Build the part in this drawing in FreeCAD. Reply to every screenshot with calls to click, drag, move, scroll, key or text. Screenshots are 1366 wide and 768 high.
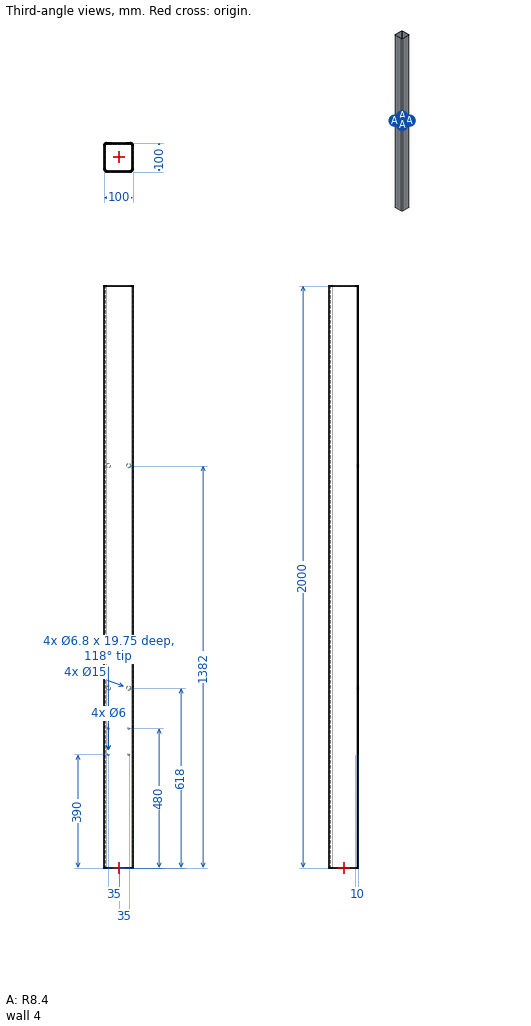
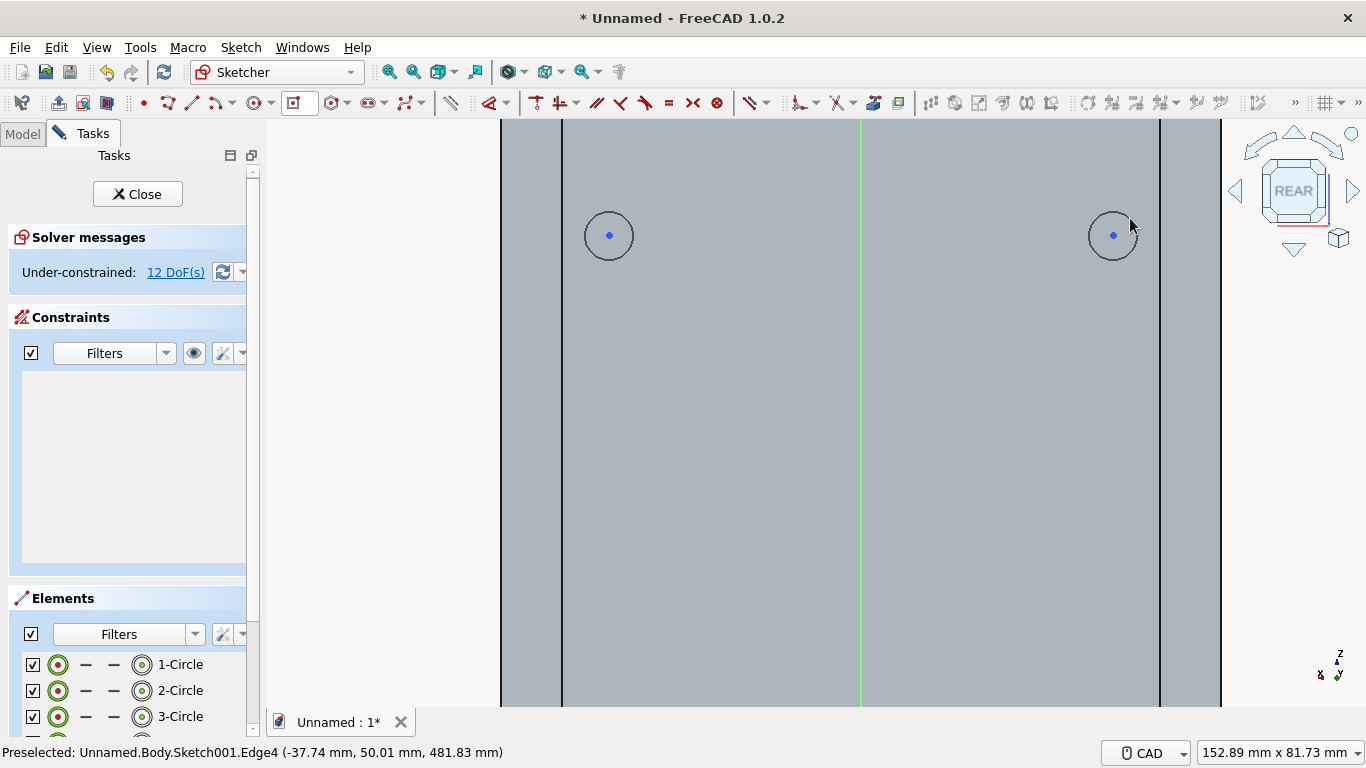
scroll(610, 236, down, 3)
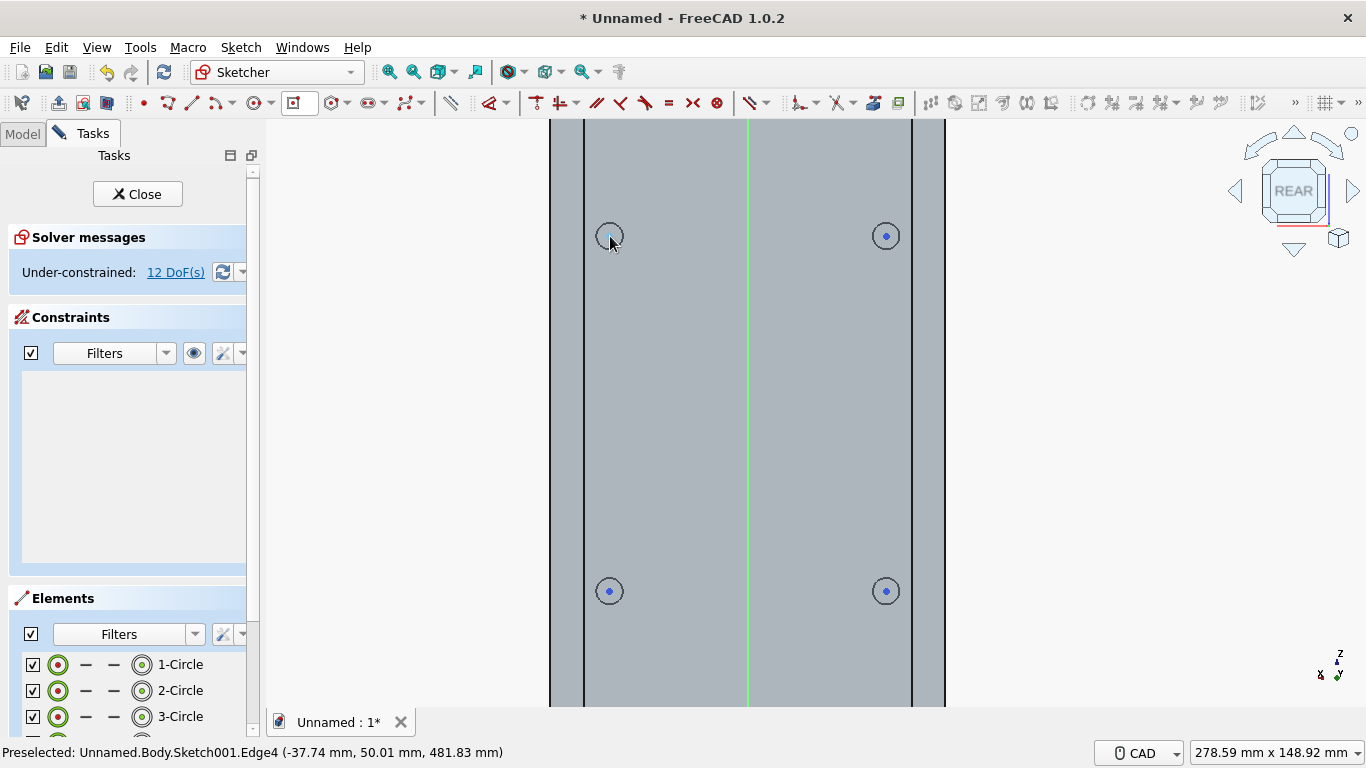
click(895, 582)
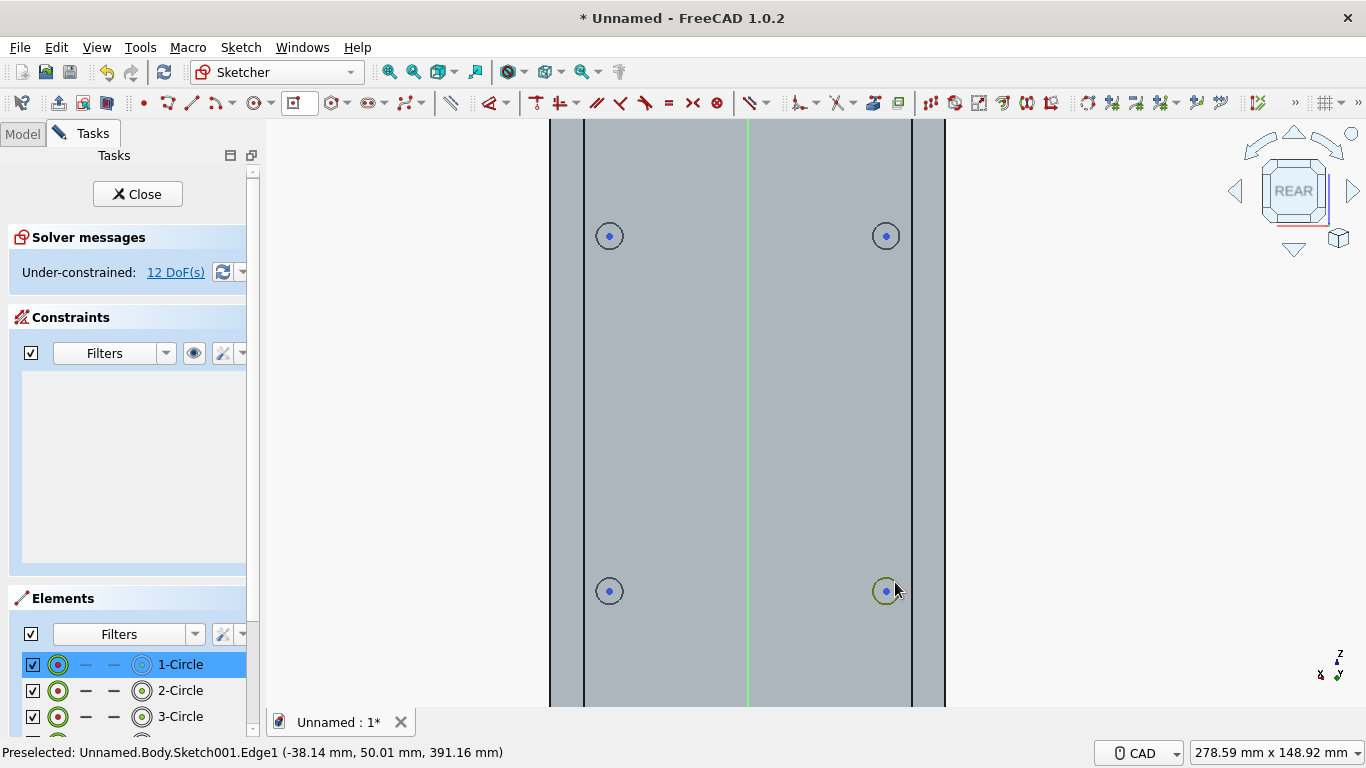
click(619, 582)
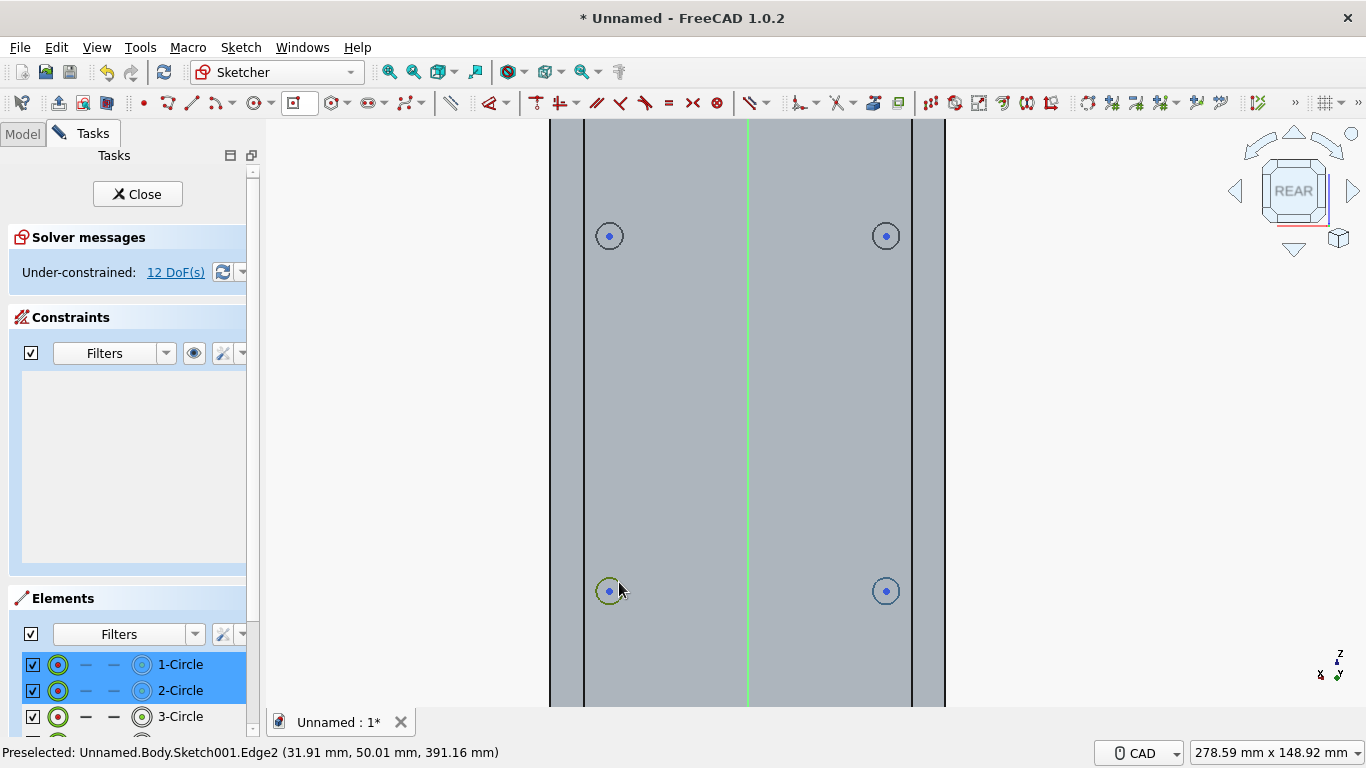
click(619, 227)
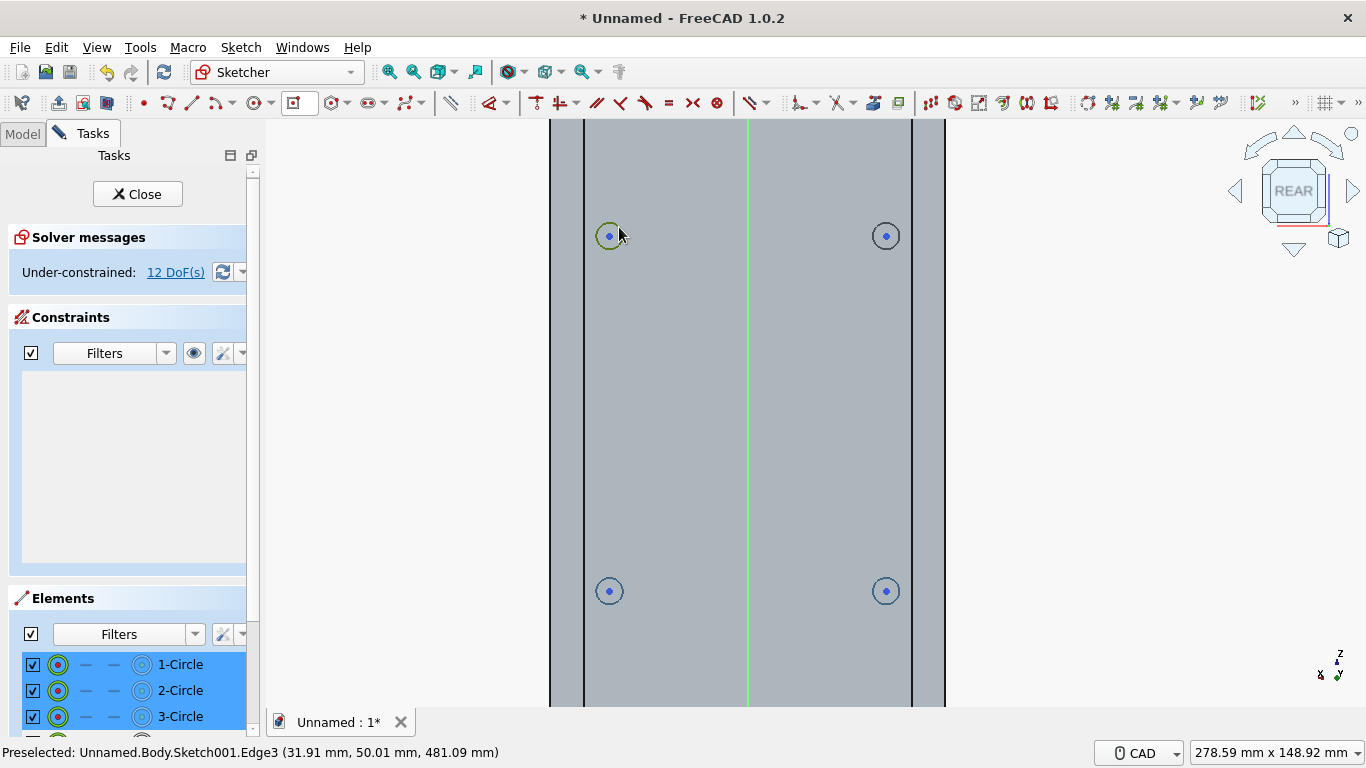
click(895, 227)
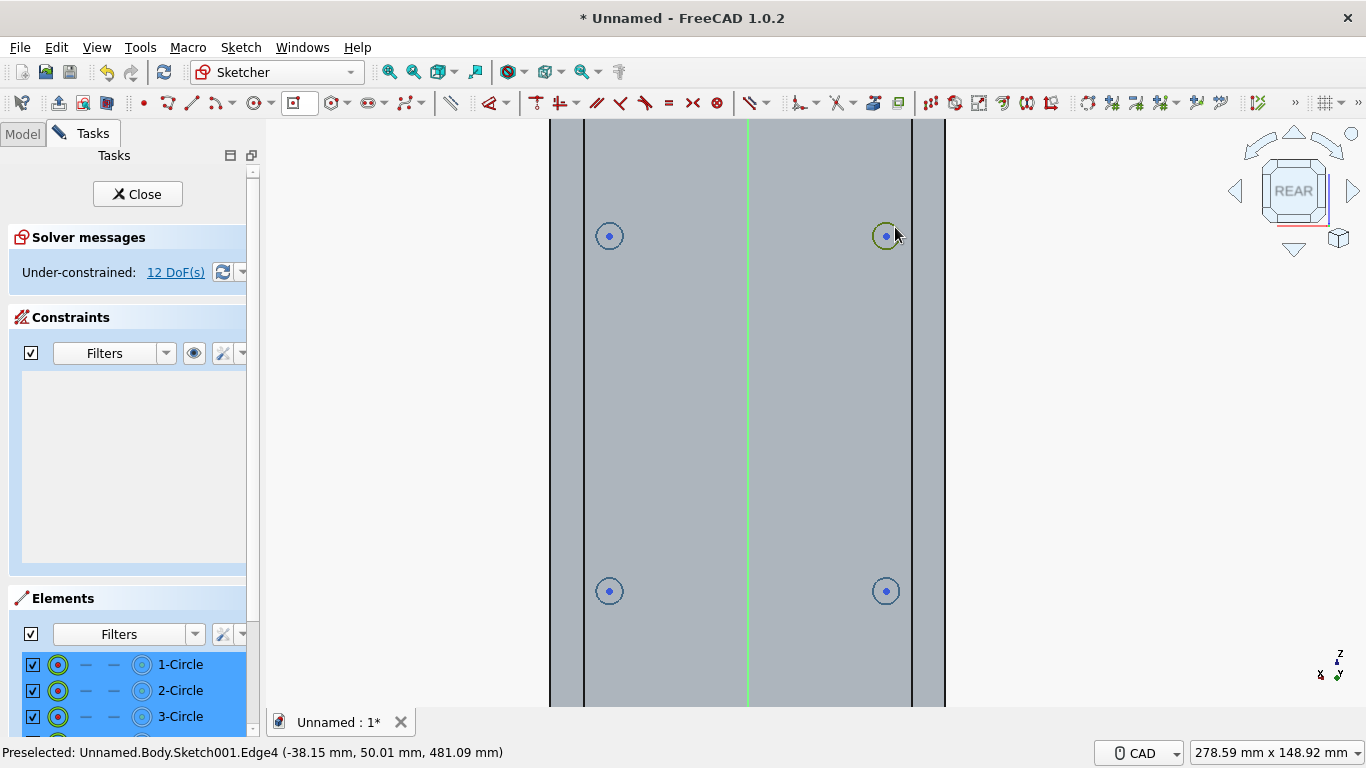
click(670, 104)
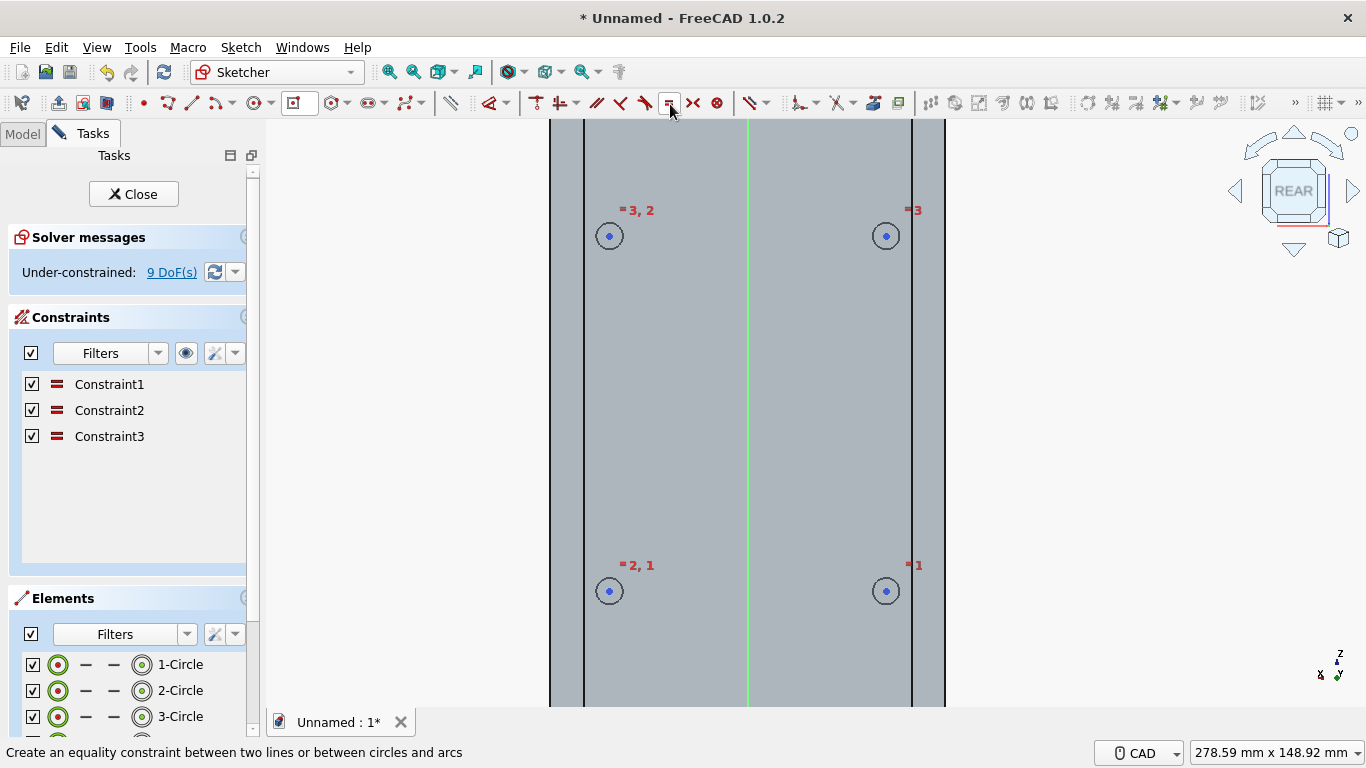
click(886, 591)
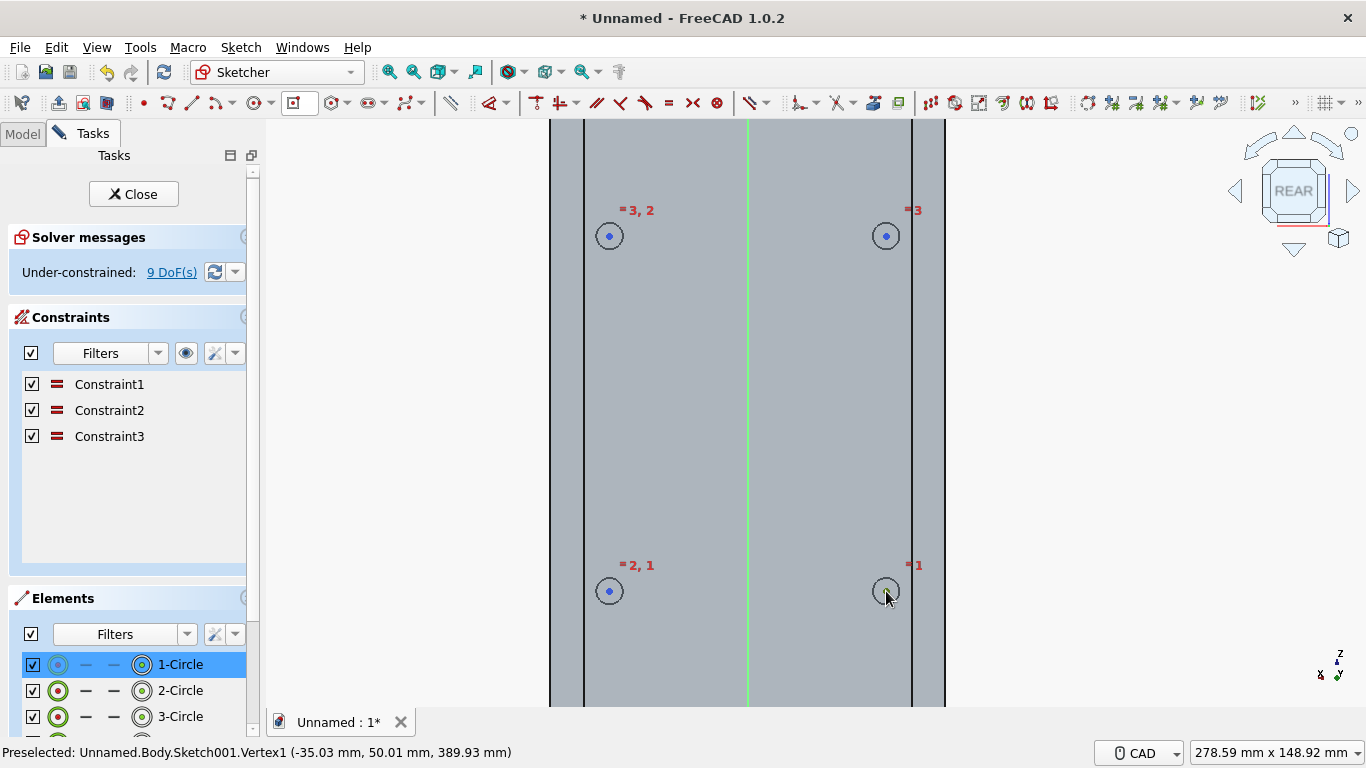
click(610, 591)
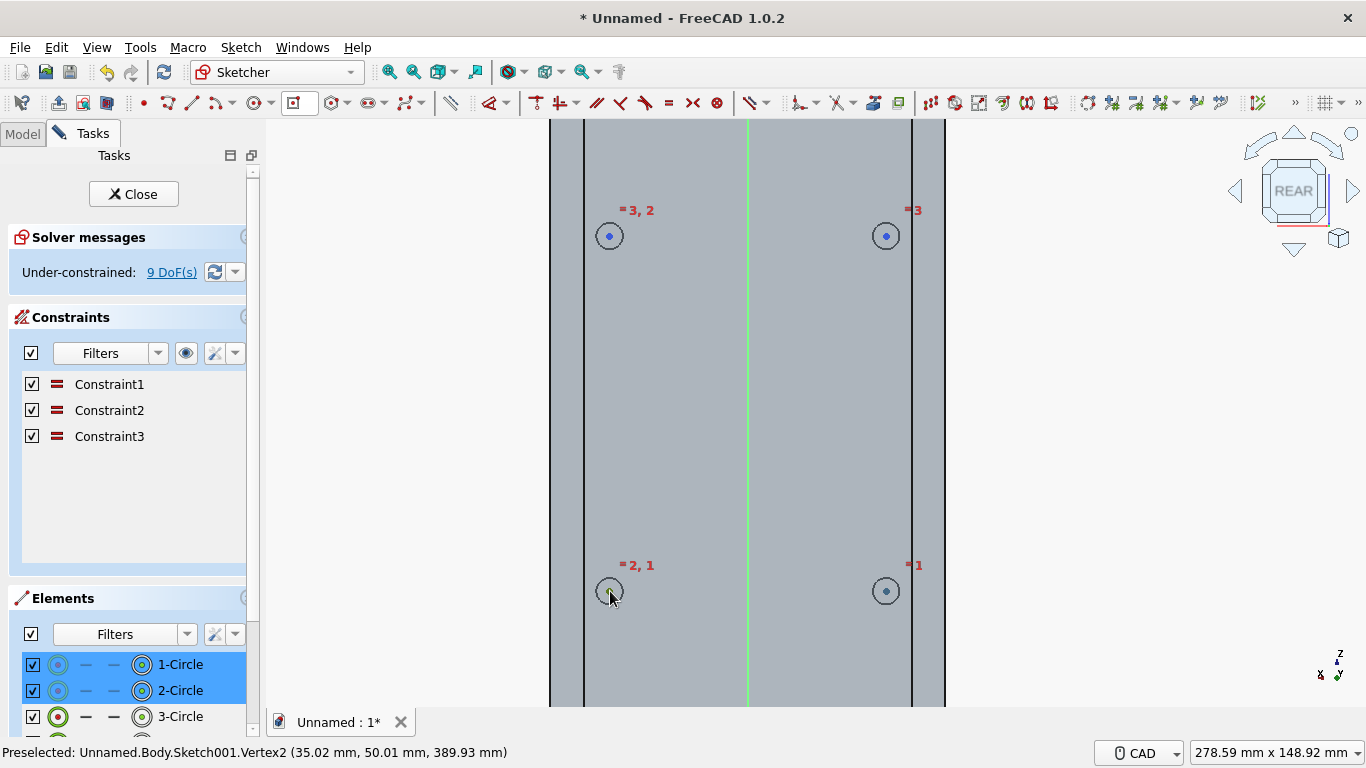
click(578, 104)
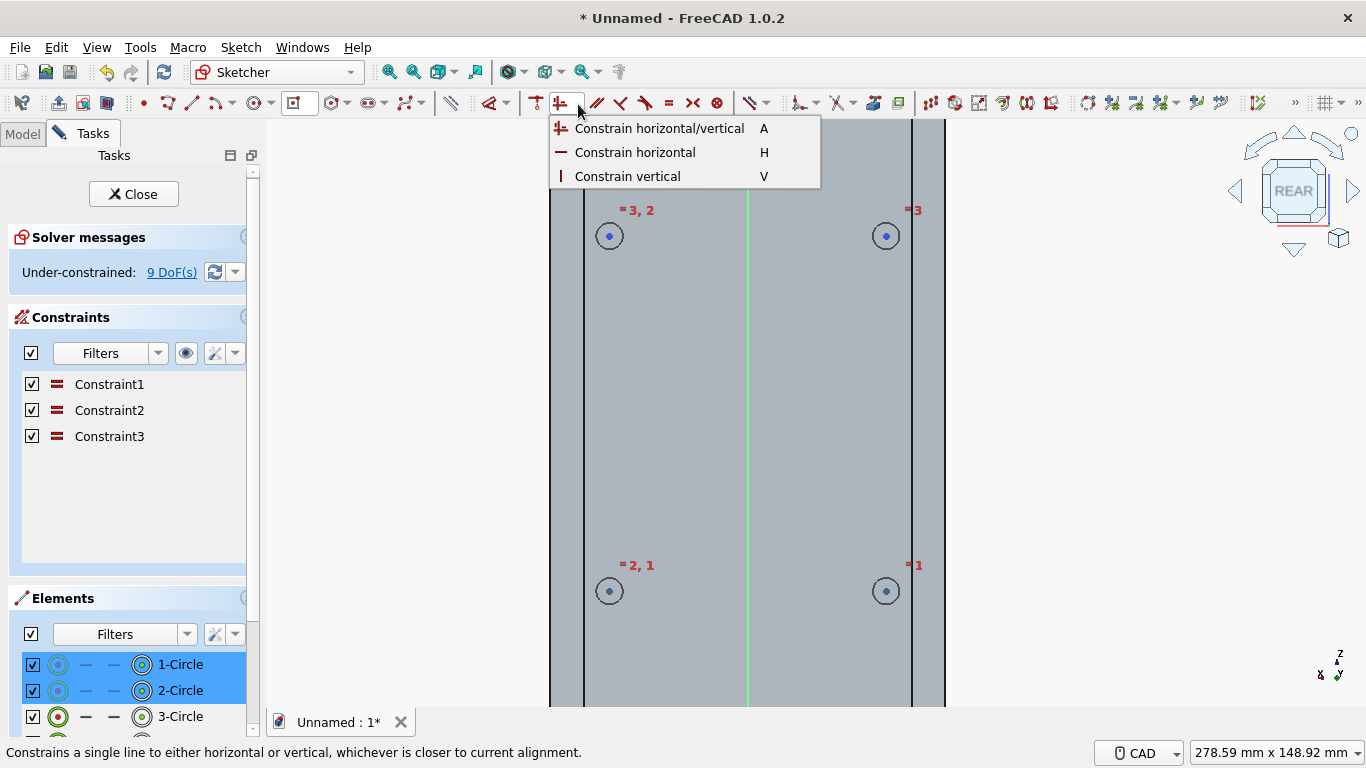
click(685, 152)